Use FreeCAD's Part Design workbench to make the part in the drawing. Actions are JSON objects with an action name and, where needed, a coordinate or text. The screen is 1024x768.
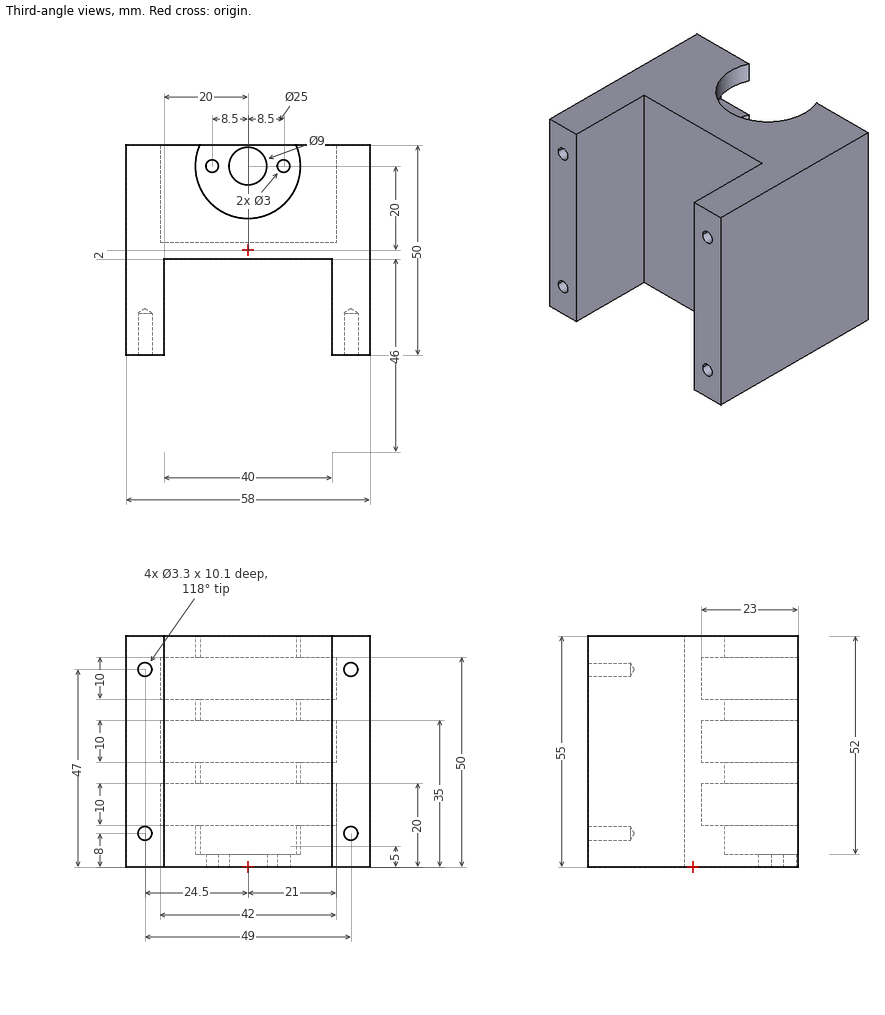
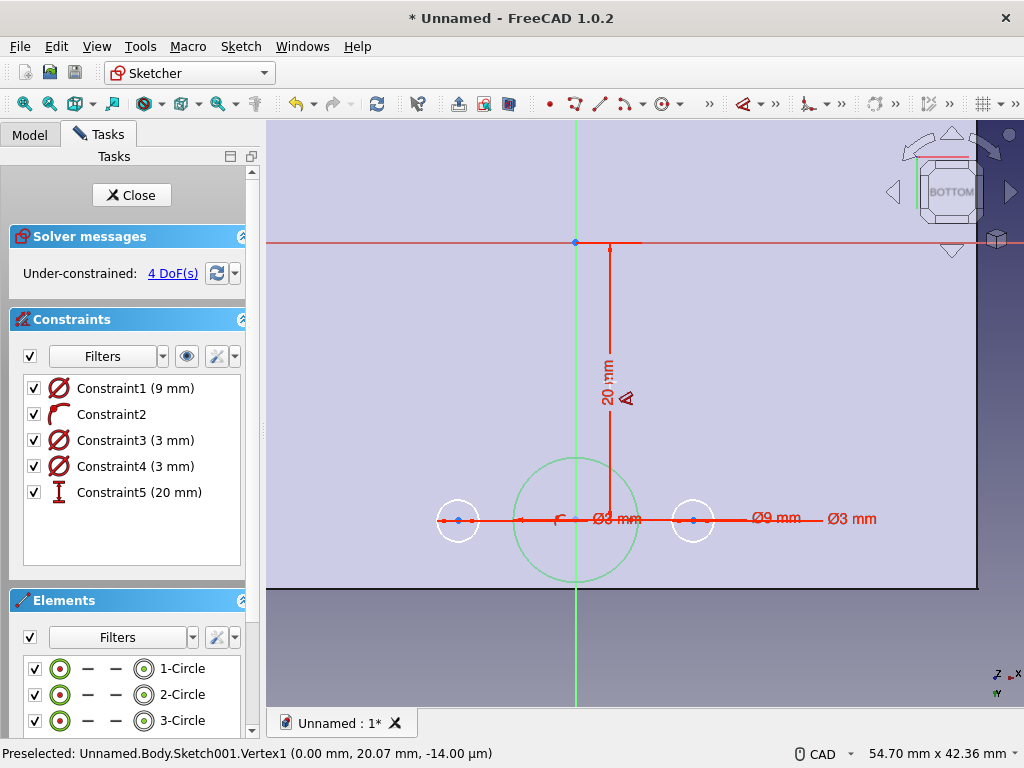
{"action": "left_click", "coordinate": [693, 521]}
{"action": "left_click", "coordinate": [727, 382]}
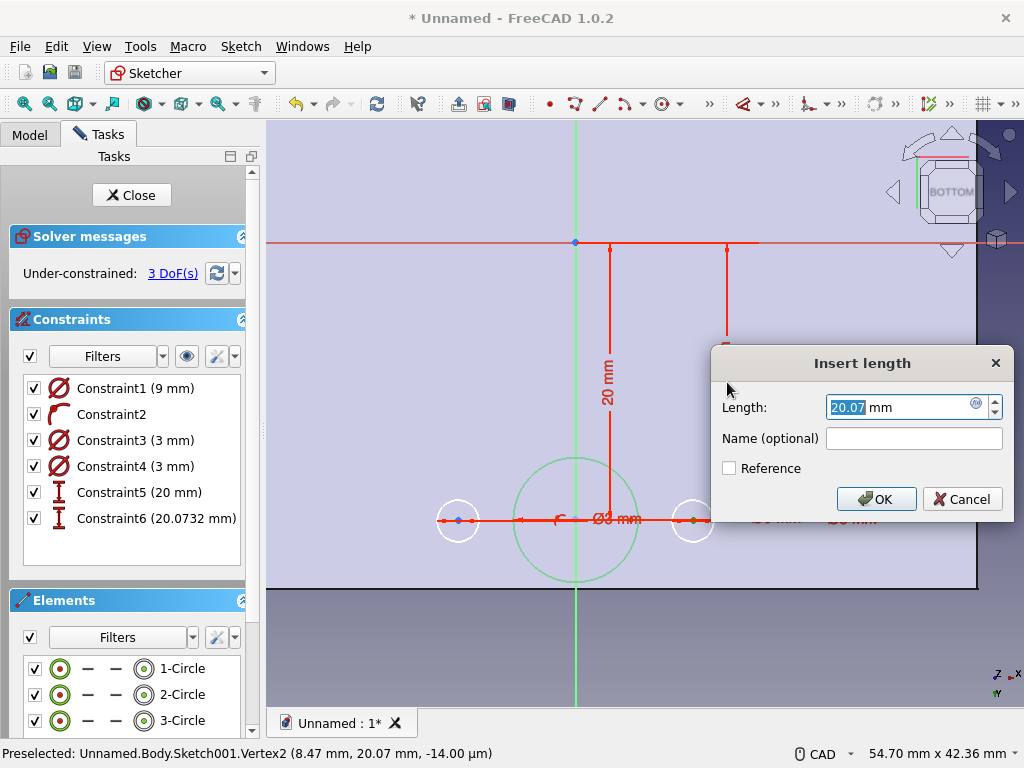
{"action": "type", "text": "20"}
{"action": "key", "text": "Return"}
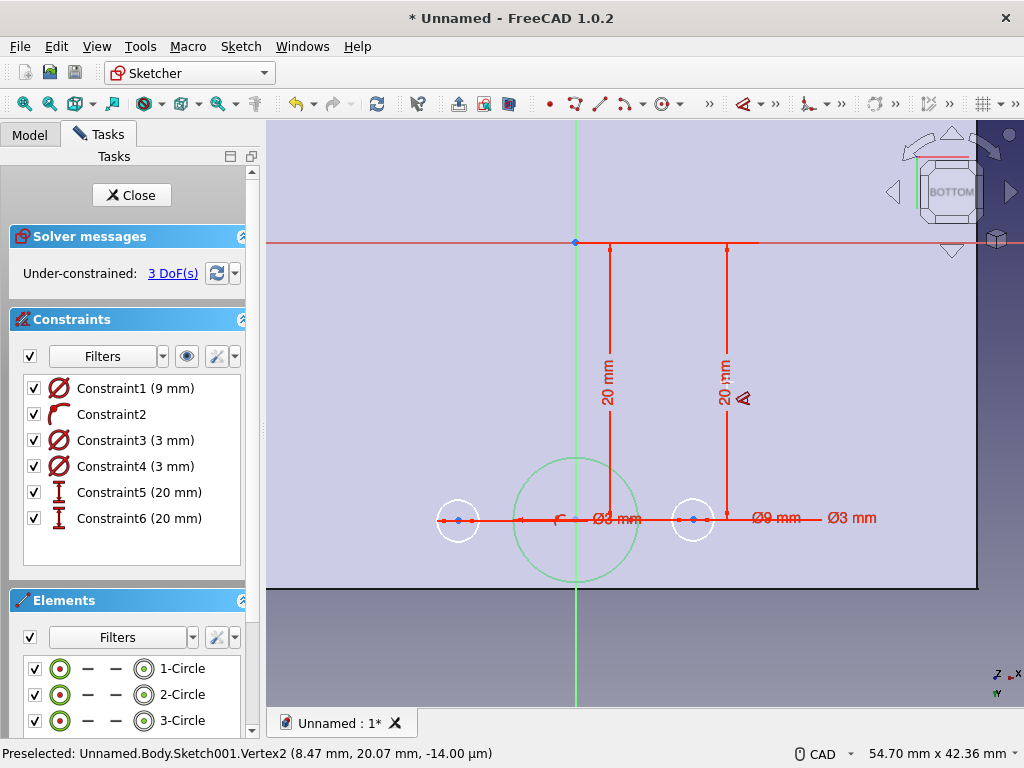
{"action": "left_click", "coordinate": [458, 521]}
{"action": "left_click", "coordinate": [424, 382]}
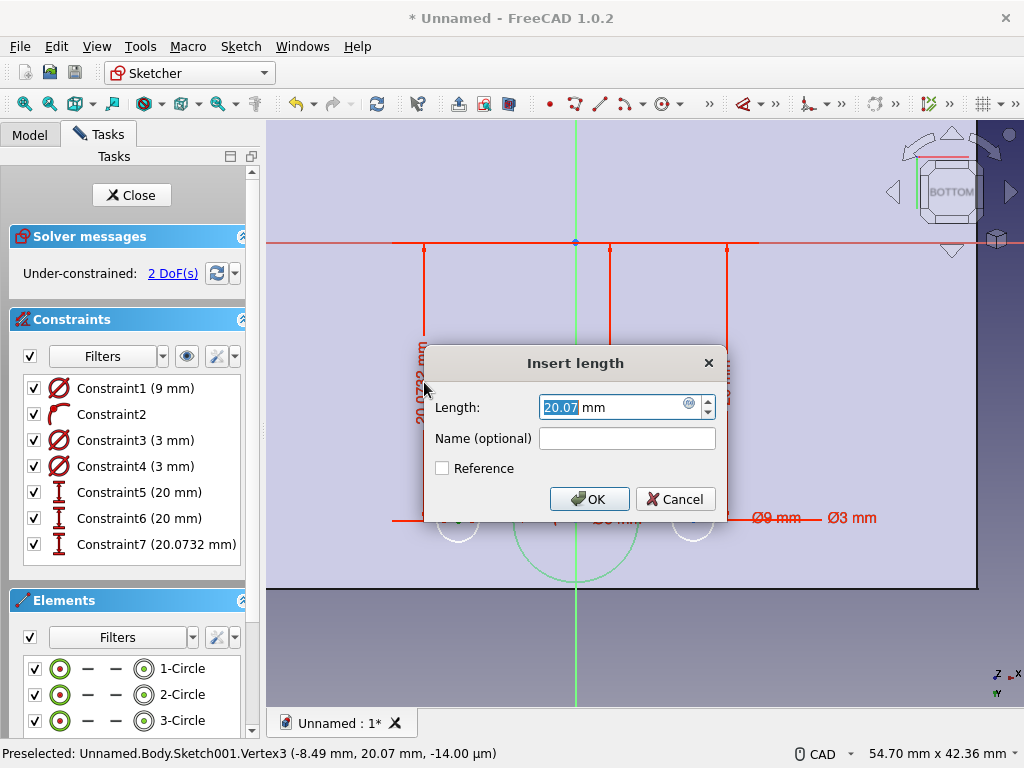
{"action": "type", "text": "20"}
{"action": "key", "text": "Return"}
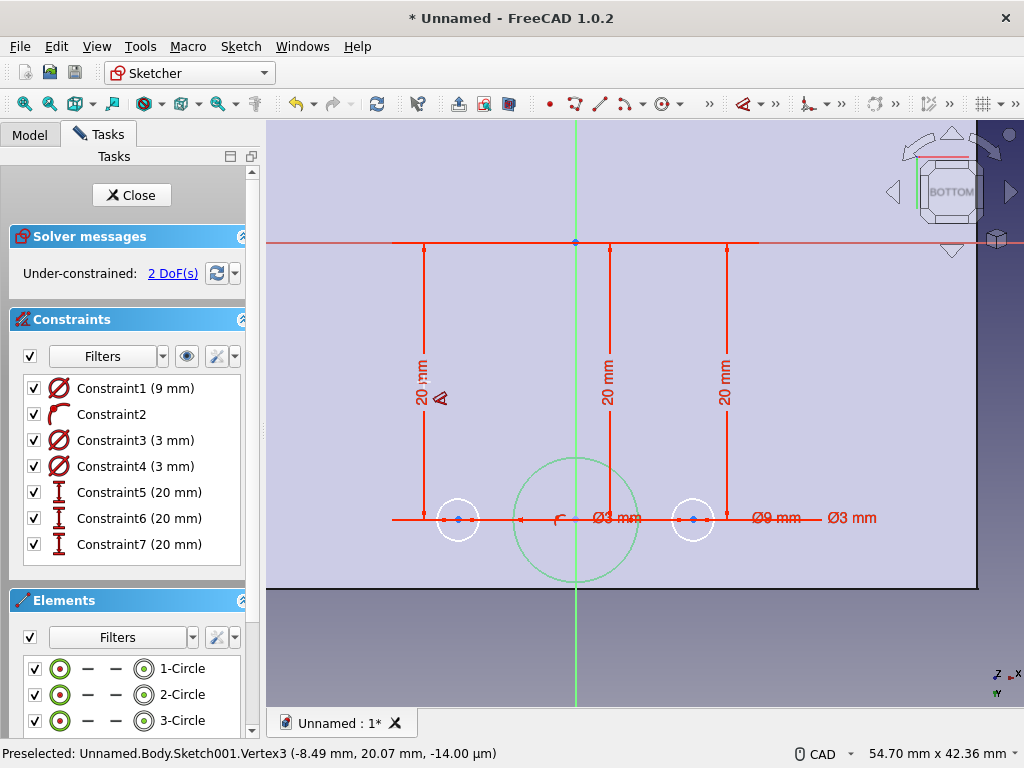
{"action": "left_click", "coordinate": [693, 520]}
{"action": "left_click", "coordinate": [634, 209]}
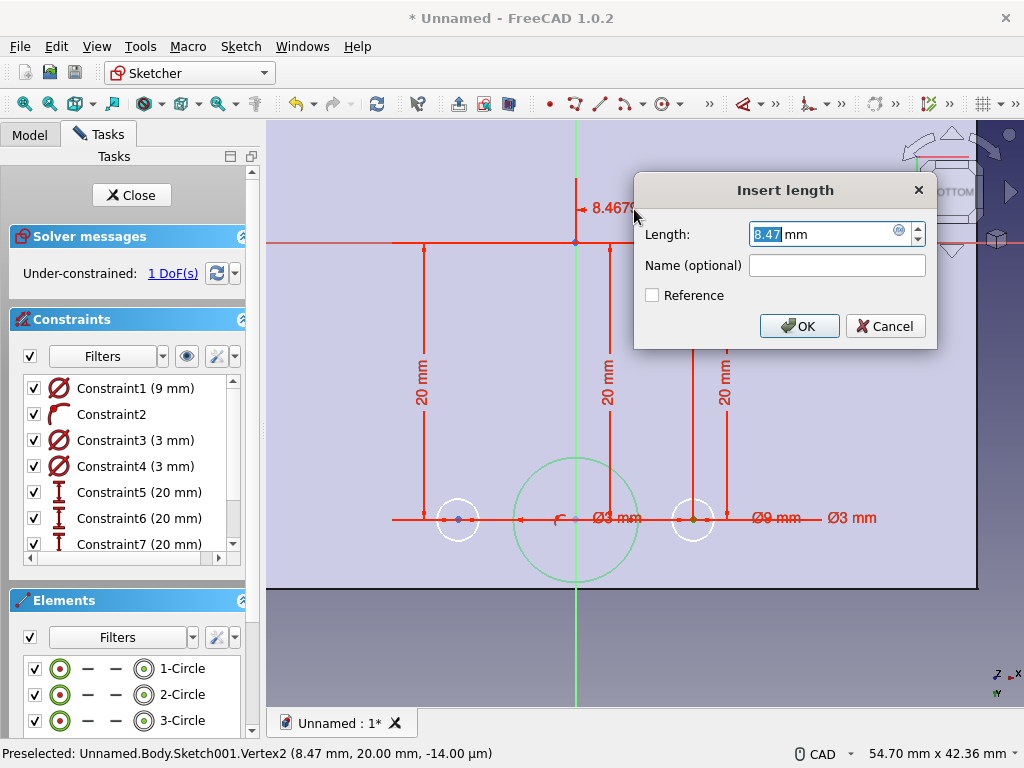
{"action": "type", "text": "8.5"}
{"action": "key", "text": "Return"}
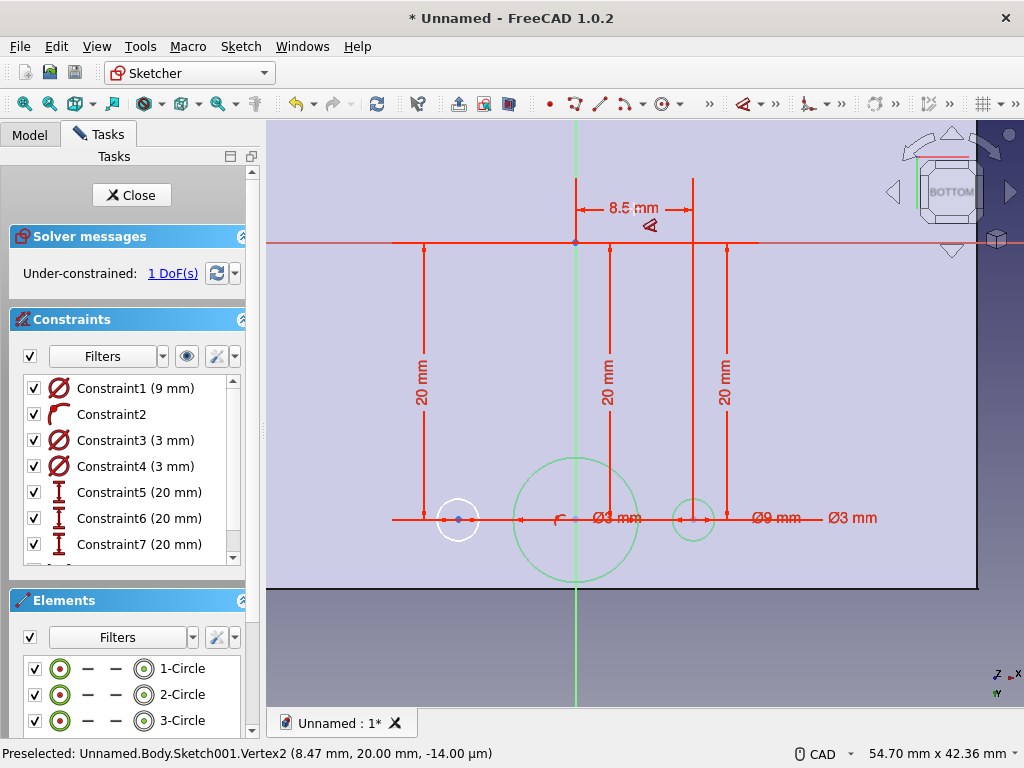
{"action": "left_click", "coordinate": [458, 520]}
{"action": "left_click", "coordinate": [517, 209]}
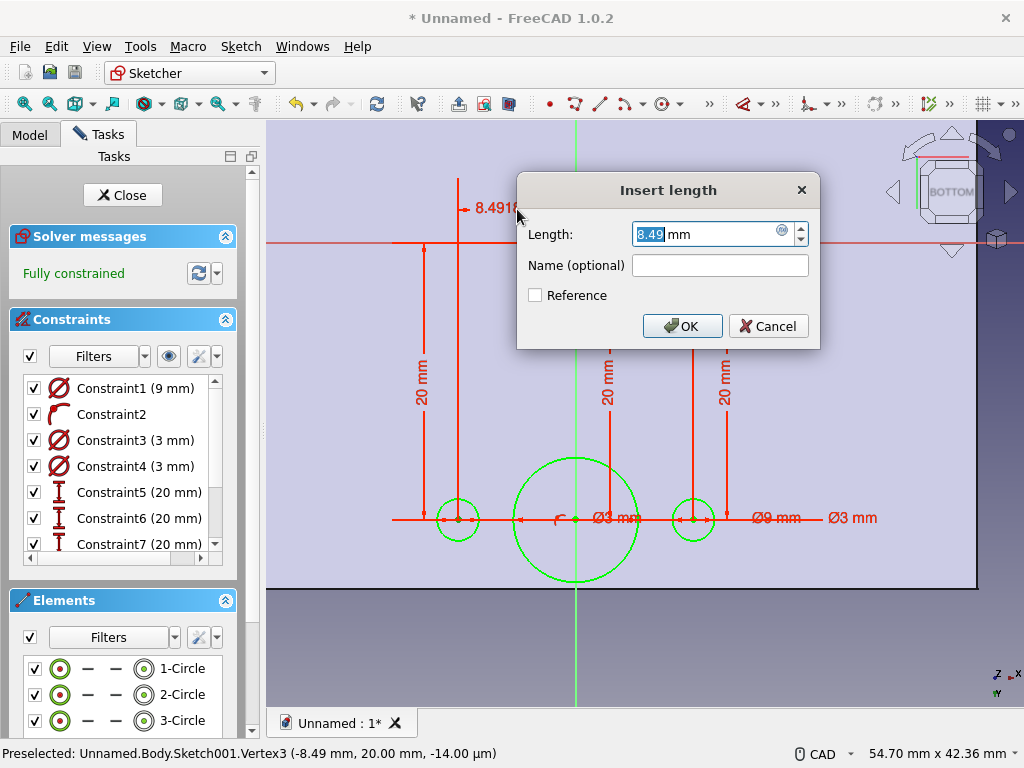
{"action": "type", "text": "8.5"}
{"action": "key", "text": "Return"}
{"action": "key", "text": "Escape"}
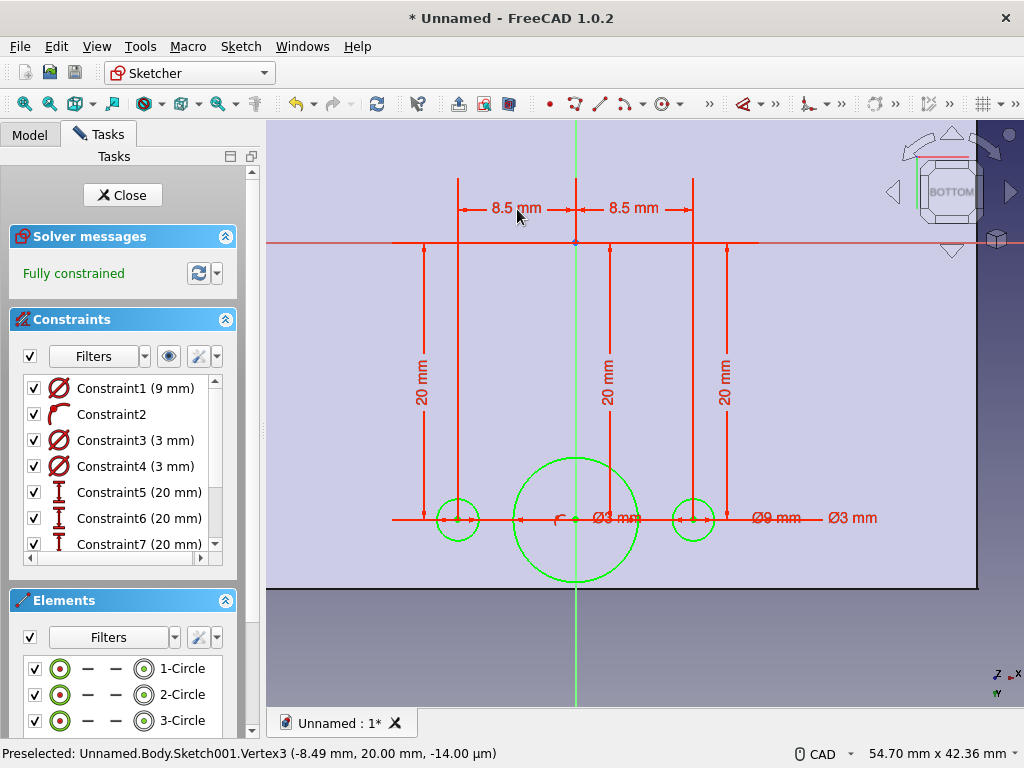
{"action": "left_click", "coordinate": [123, 195]}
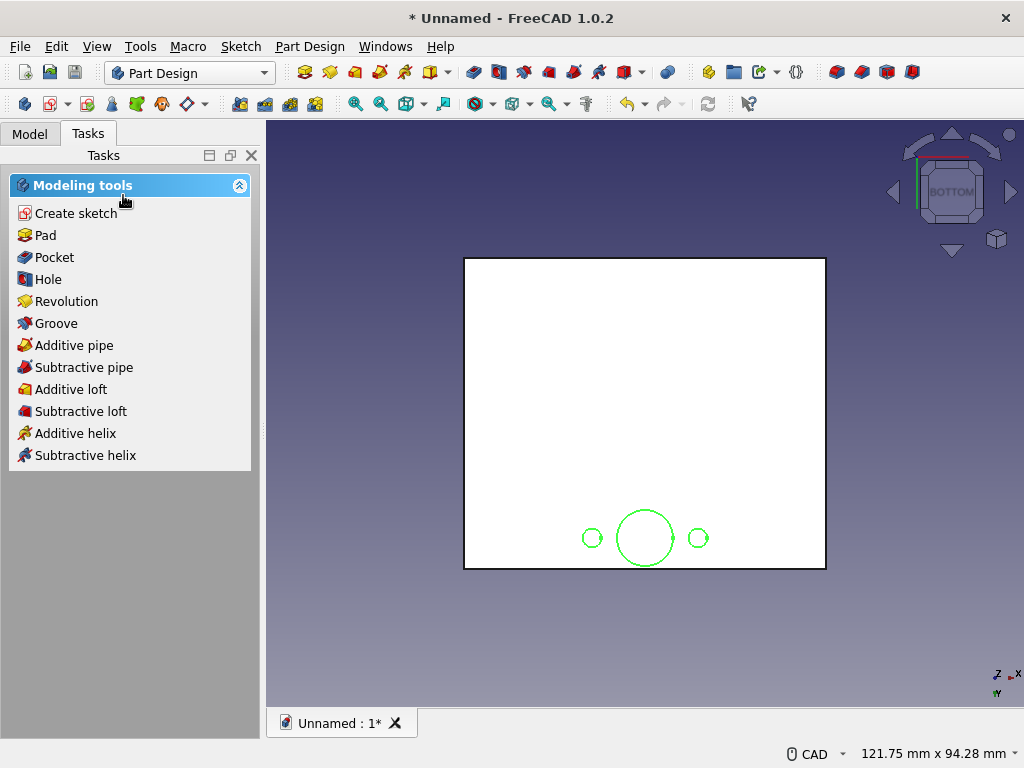
{"action": "left_click", "coordinate": [474, 72]}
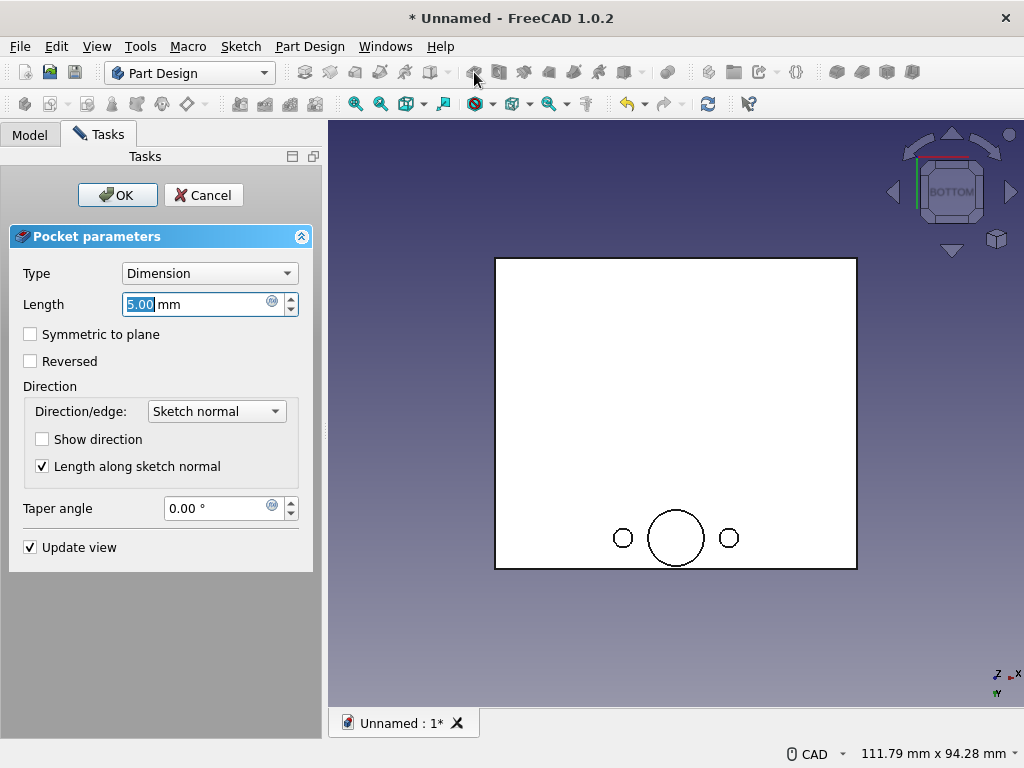
{"action": "type", "text": "5"}
{"action": "key", "text": "Tab"}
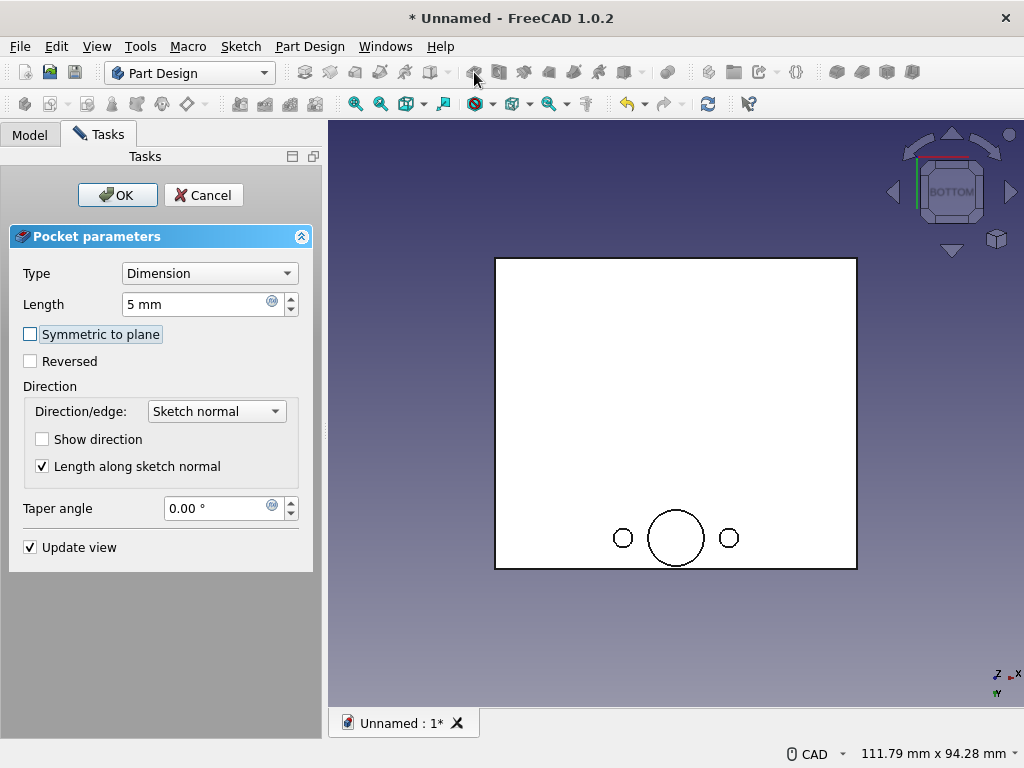
{"action": "left_click", "coordinate": [118, 195]}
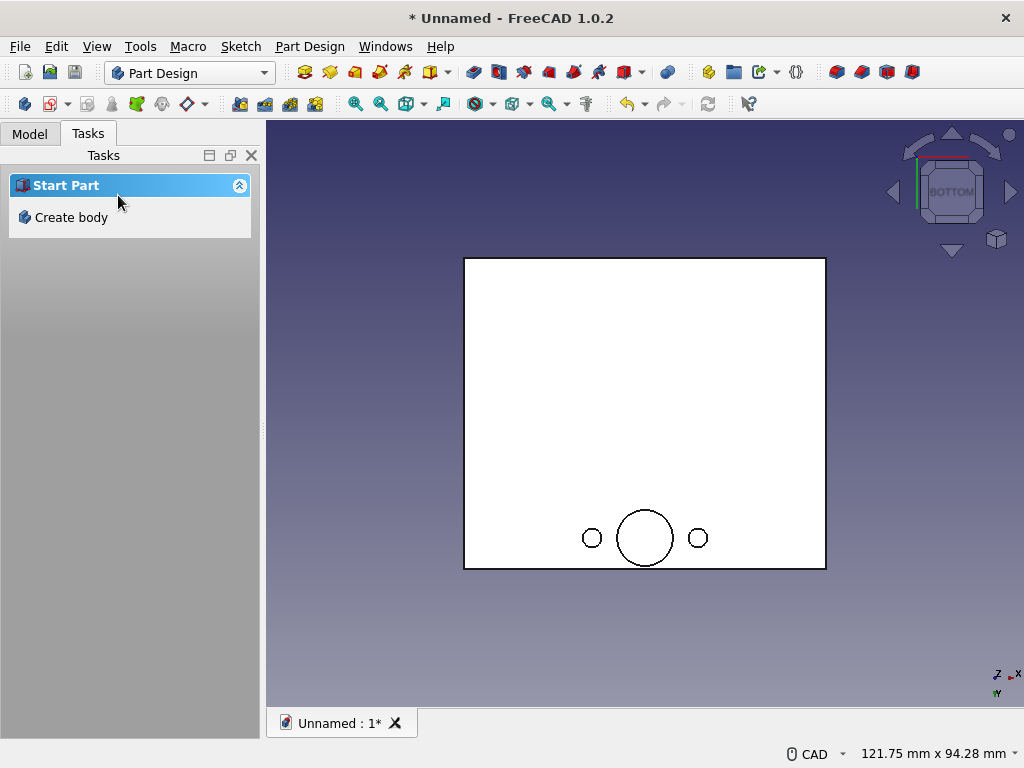
{"action": "key", "text": "0"}